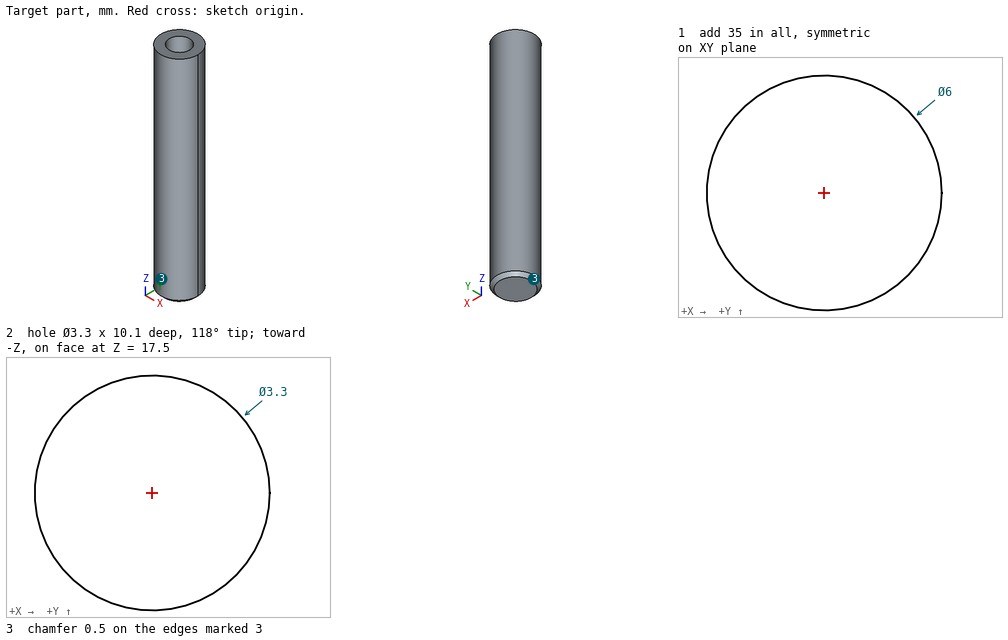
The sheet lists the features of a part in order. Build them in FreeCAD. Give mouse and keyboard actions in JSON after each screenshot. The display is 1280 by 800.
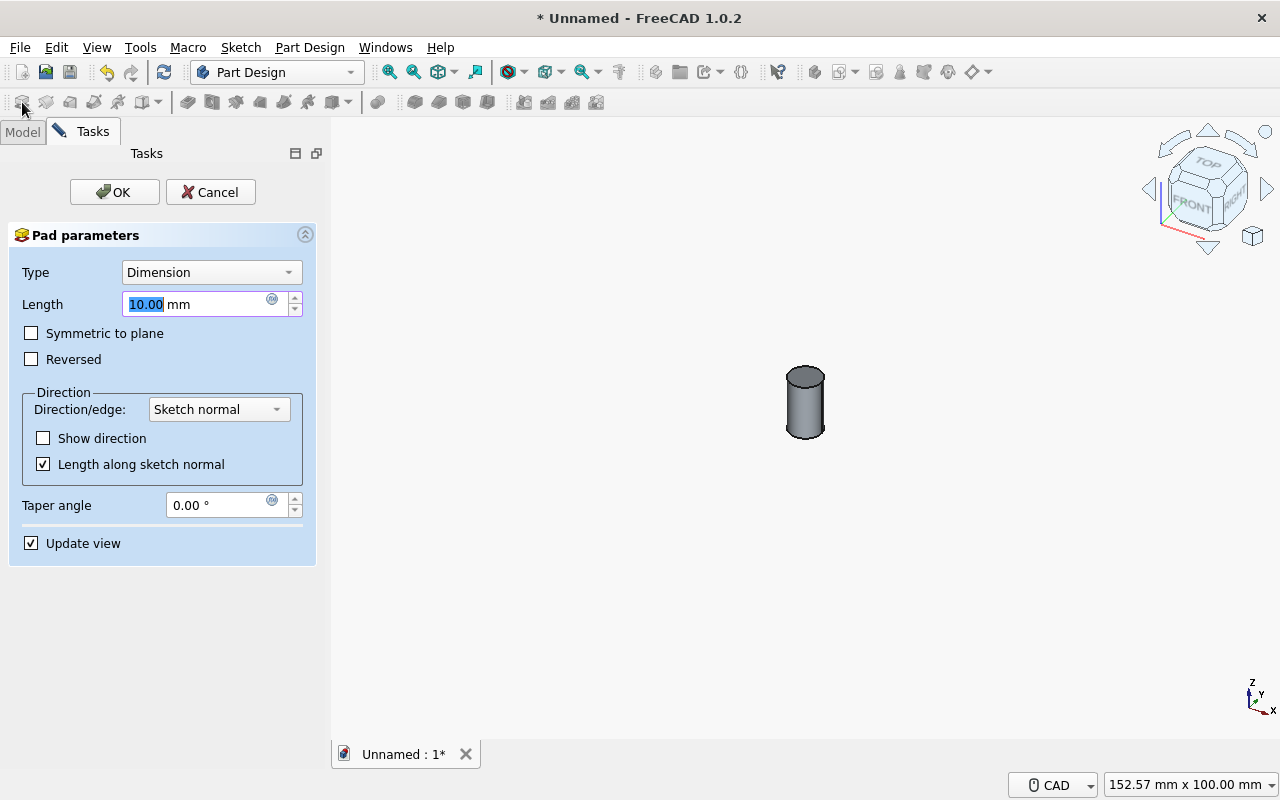
{"action": "type", "text": "35"}
{"action": "key", "text": "Tab"}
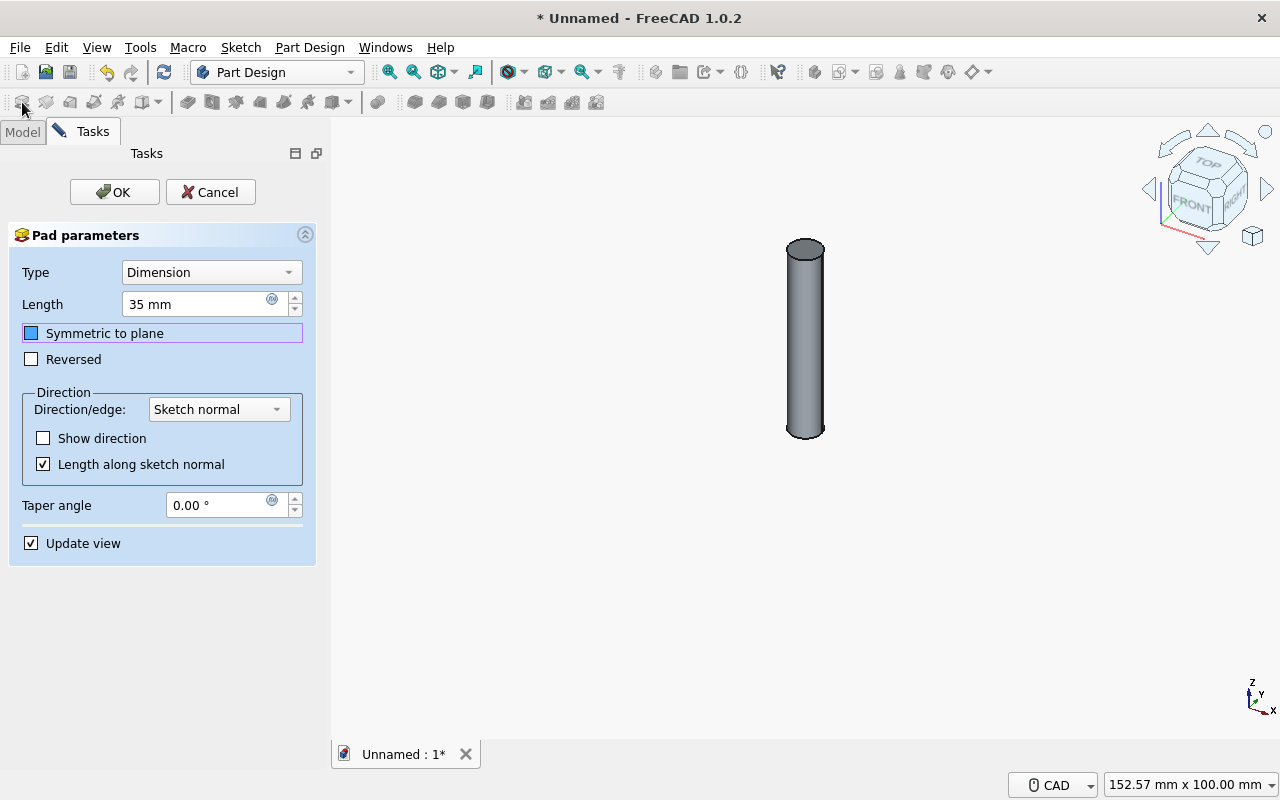
{"action": "left_click", "coordinate": [30, 333]}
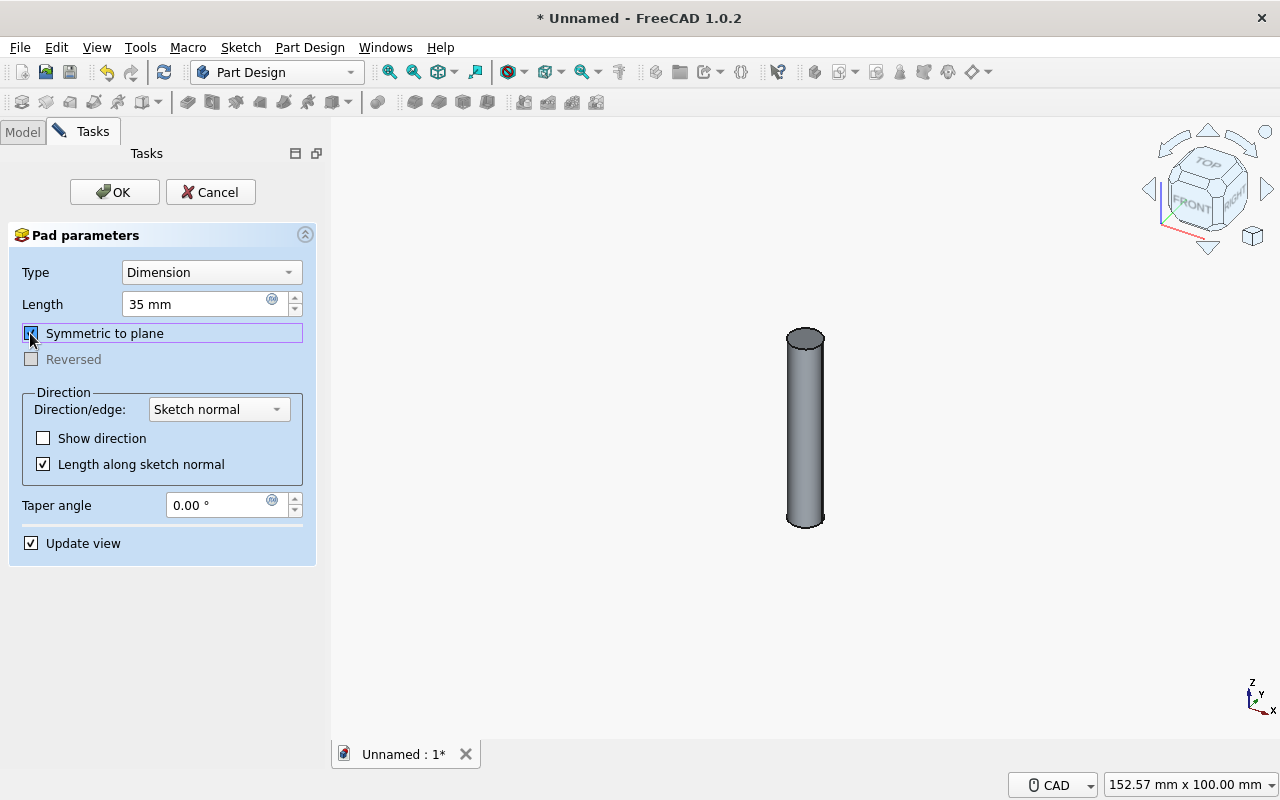
{"action": "left_click", "coordinate": [115, 192]}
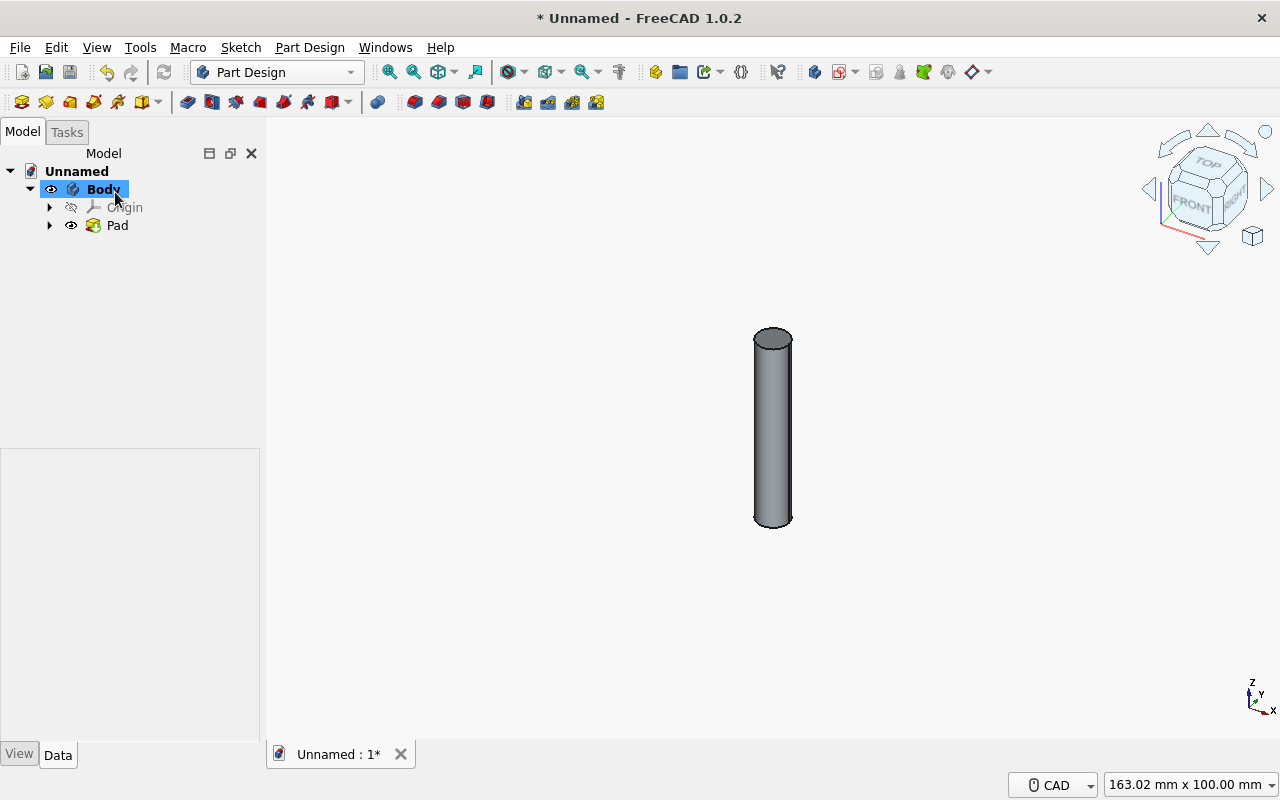
{"action": "left_click", "coordinate": [390, 72]}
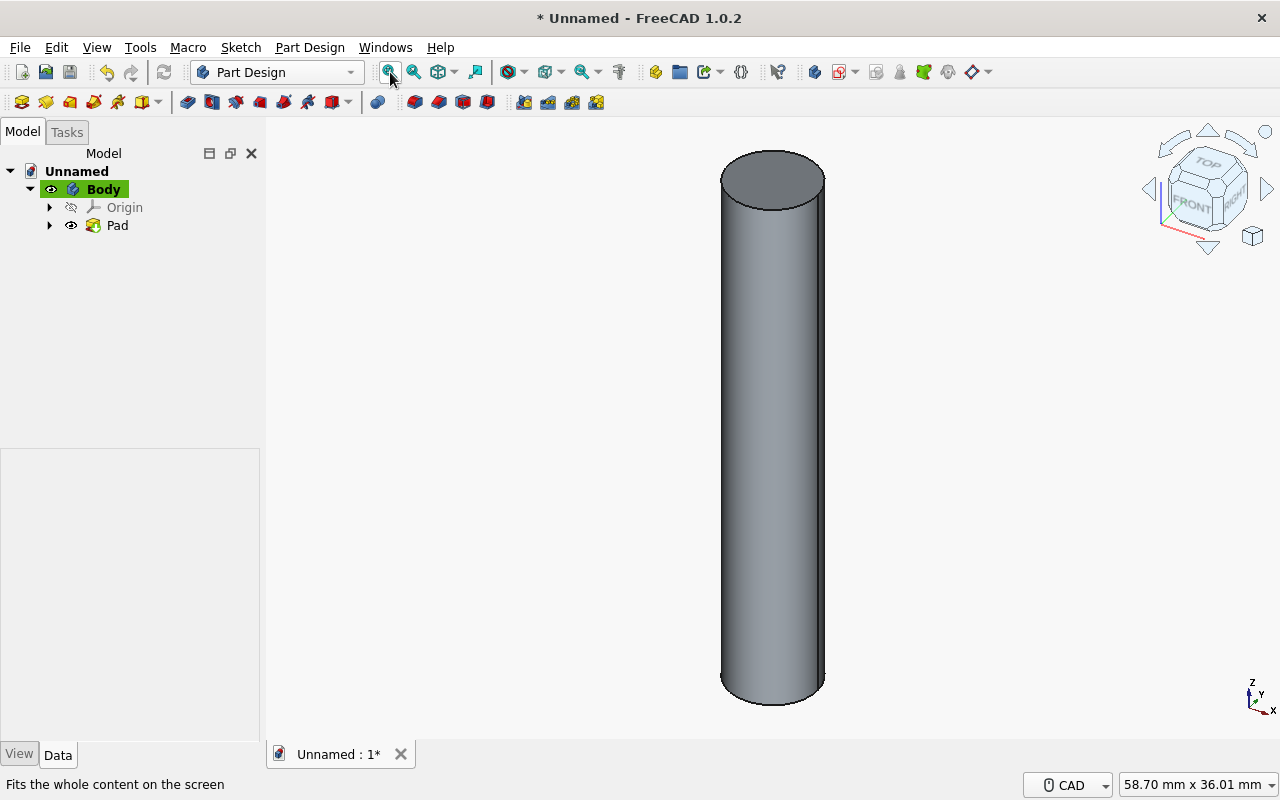
{"action": "left_click", "coordinate": [773, 179]}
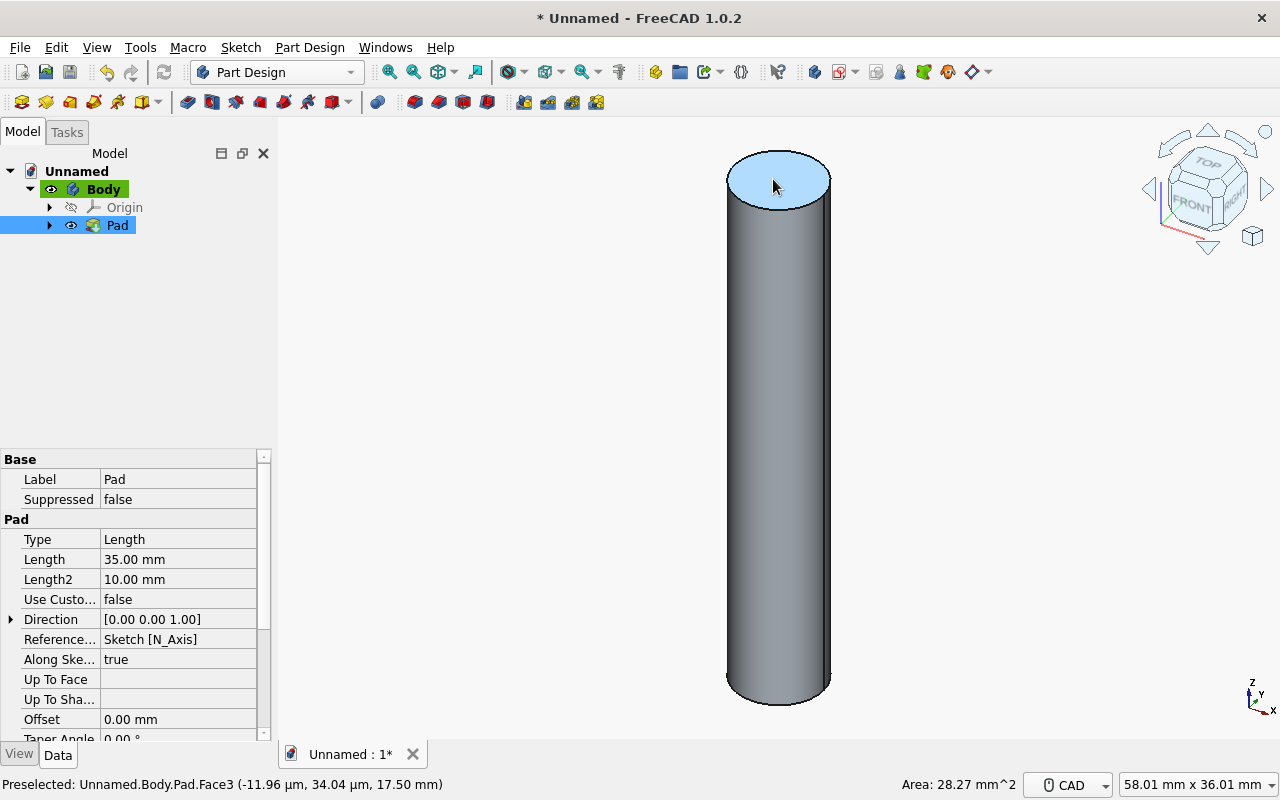
{"action": "left_click", "coordinate": [840, 72]}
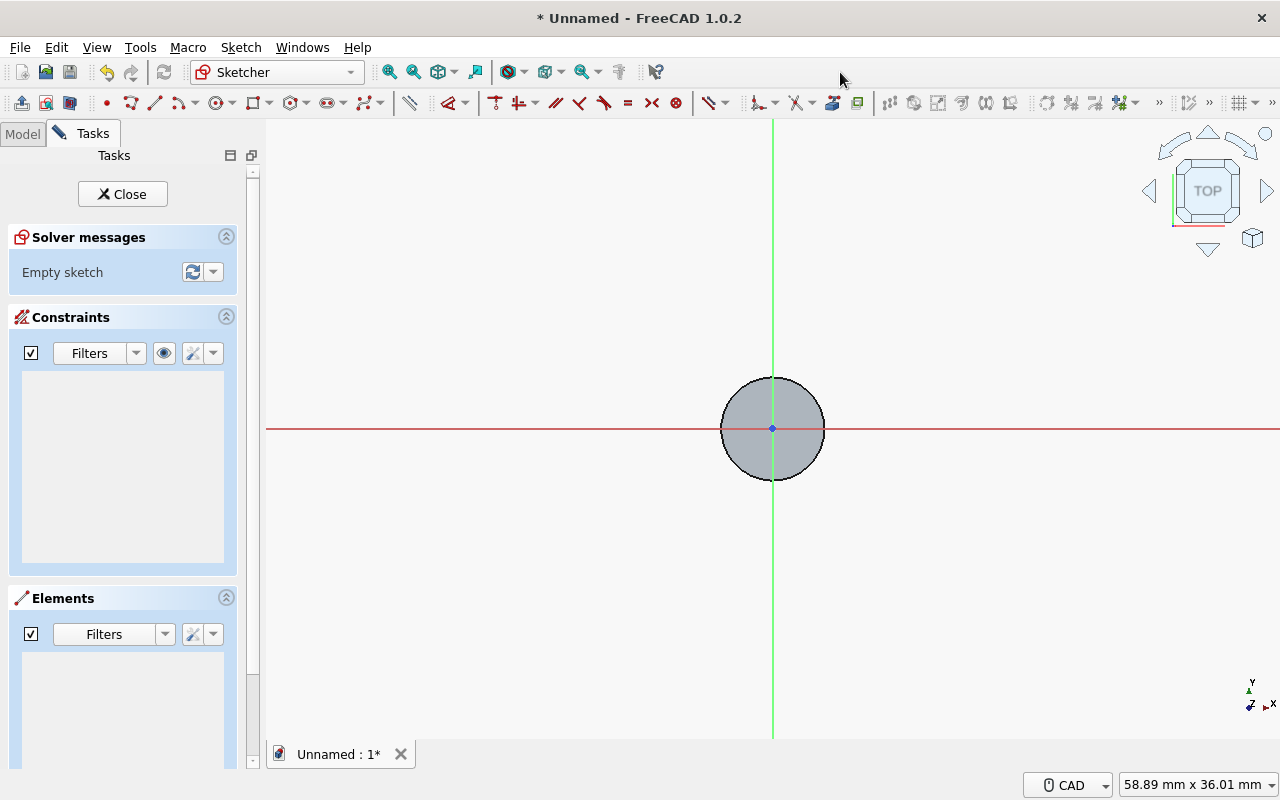
{"action": "scroll", "coordinate": [784, 429], "scroll_direction": "up", "scroll_amount": 10}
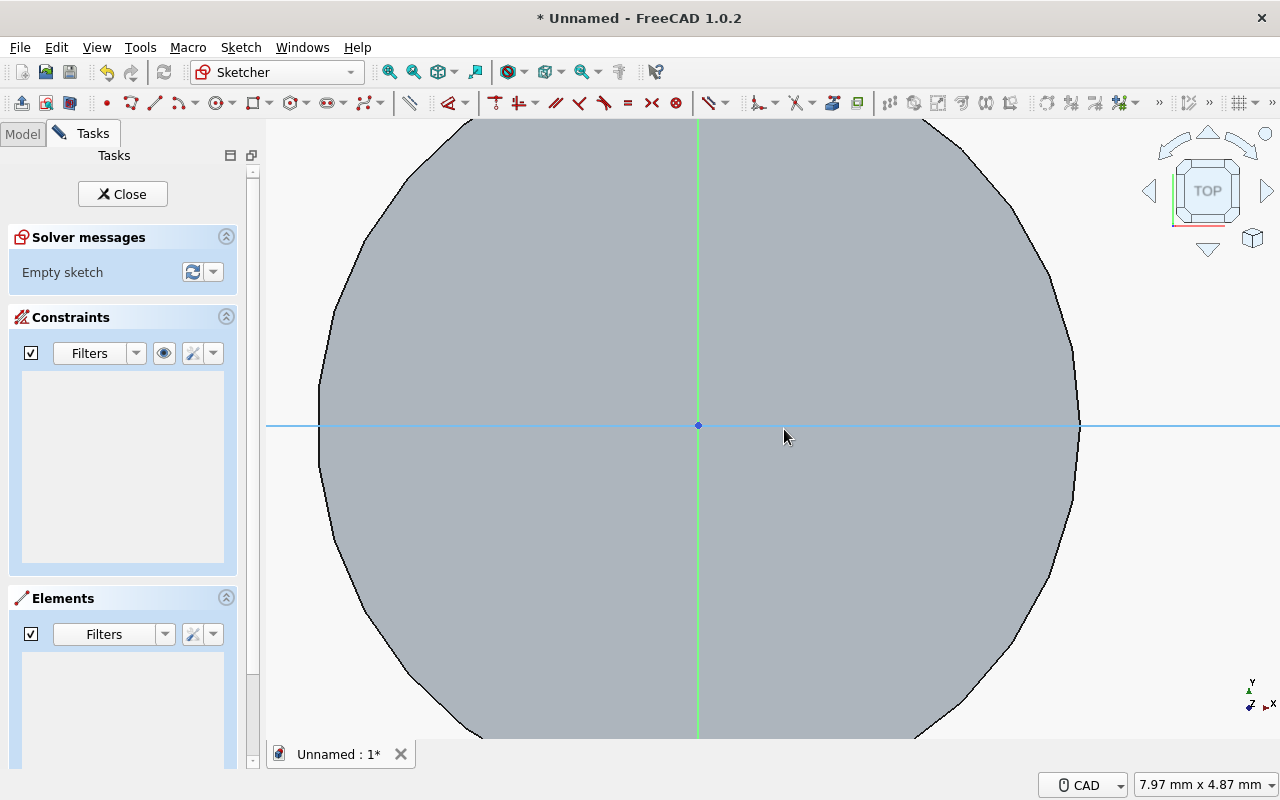
{"action": "left_click", "coordinate": [216, 104]}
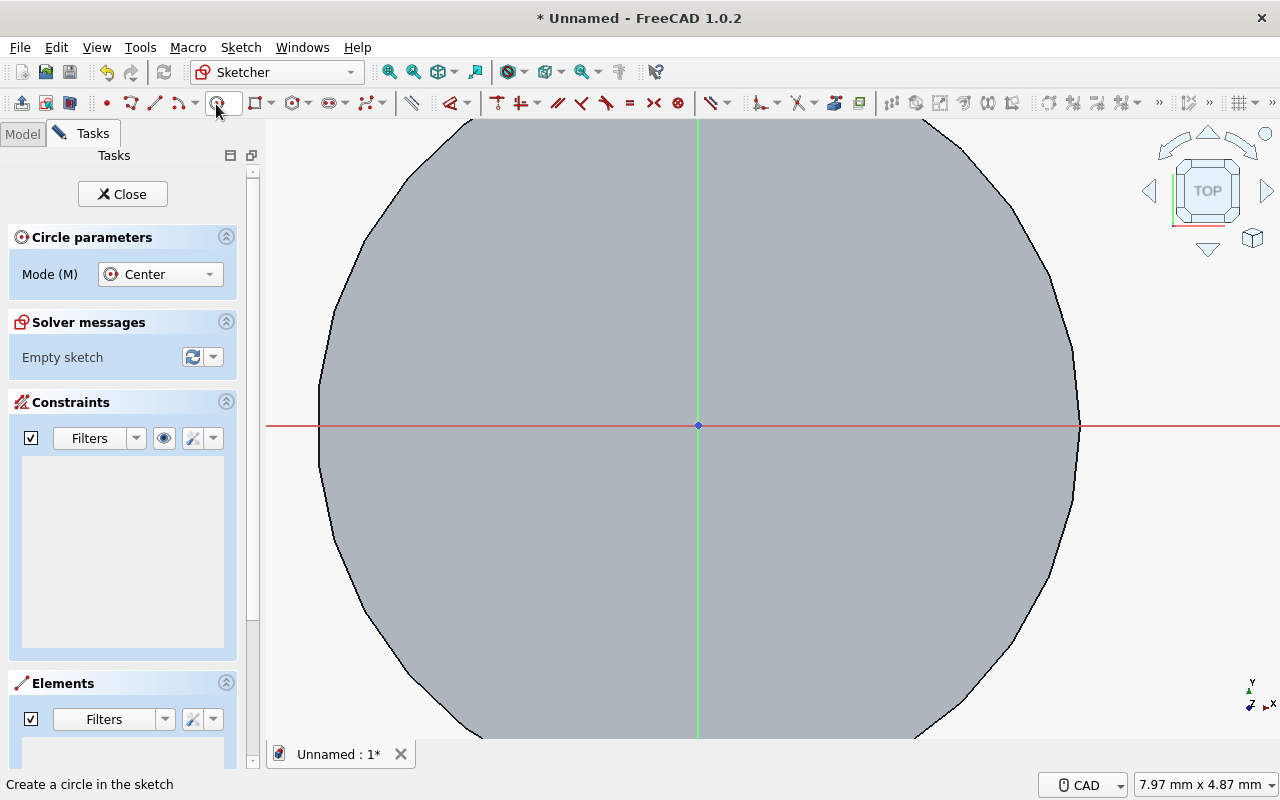
{"action": "left_click", "coordinate": [698, 426]}
{"action": "mouse_move", "coordinate": [847, 277]}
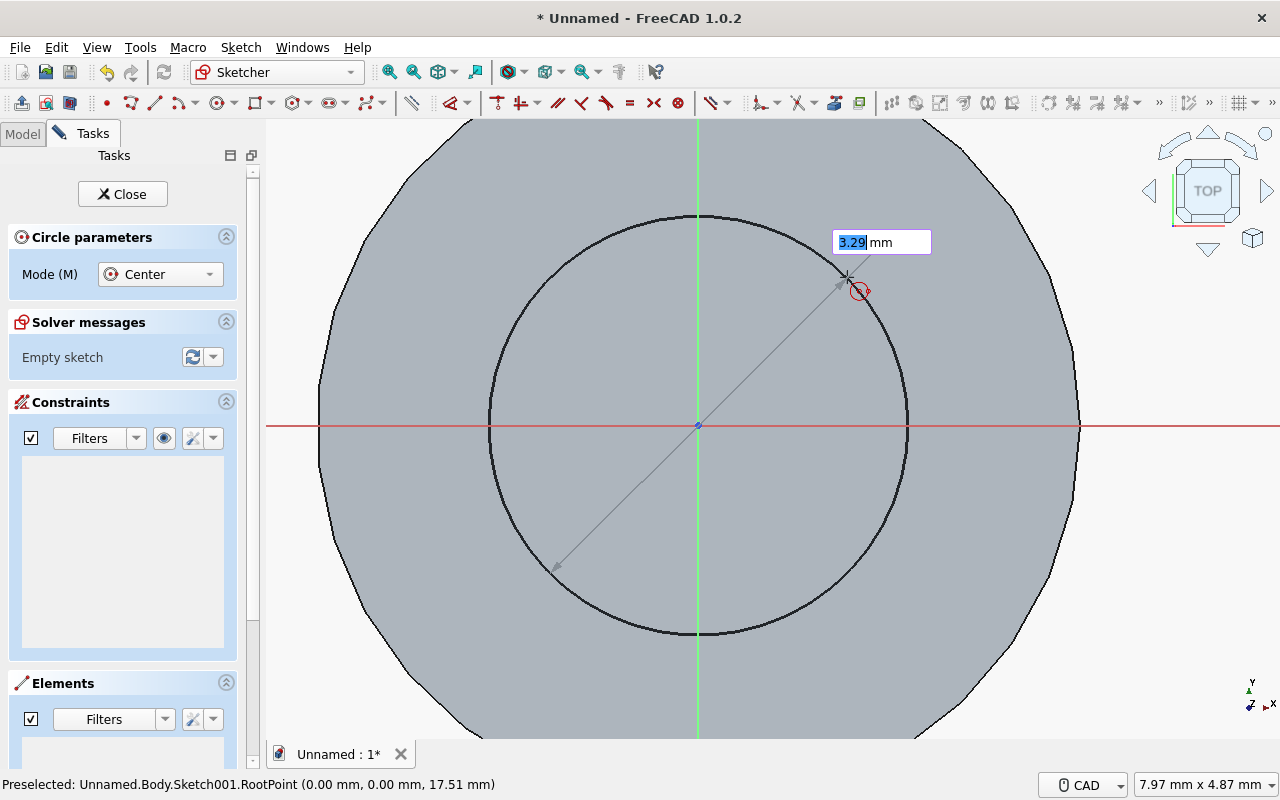
{"action": "type", "text": "3.3"}
{"action": "key", "text": "Return"}
{"action": "key", "text": "Escape"}